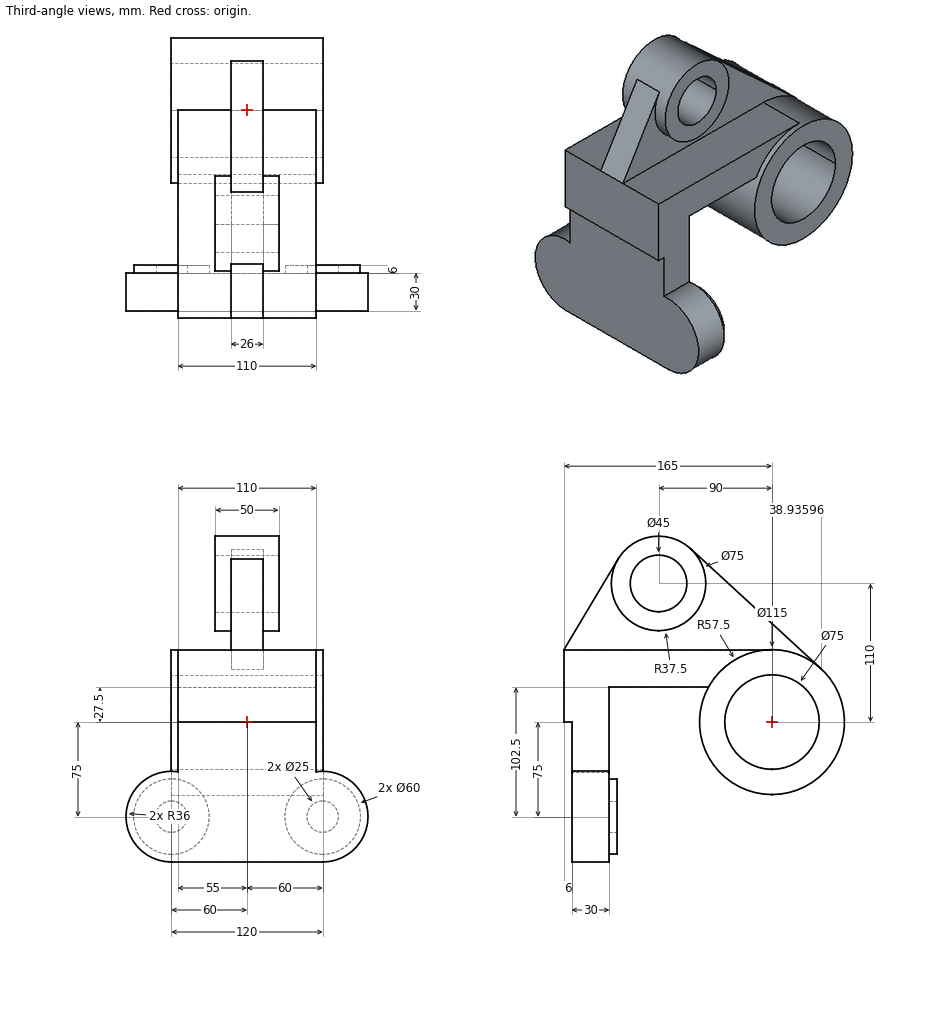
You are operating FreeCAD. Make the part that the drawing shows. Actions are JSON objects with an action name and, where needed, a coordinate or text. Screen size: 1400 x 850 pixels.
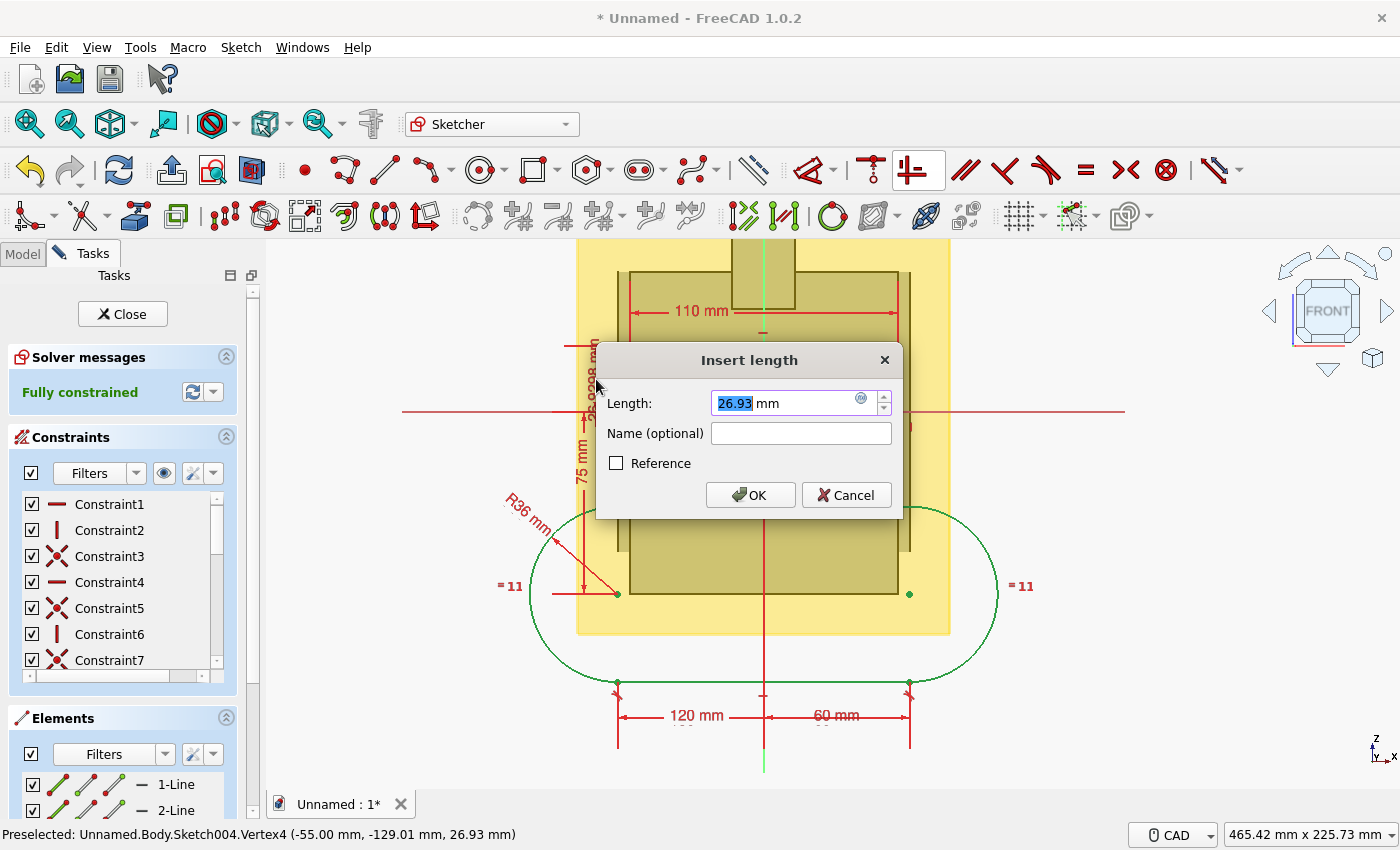
{"action": "type", "text": "27.5"}
{"action": "key", "text": "Return"}
{"action": "key", "text": "Escape"}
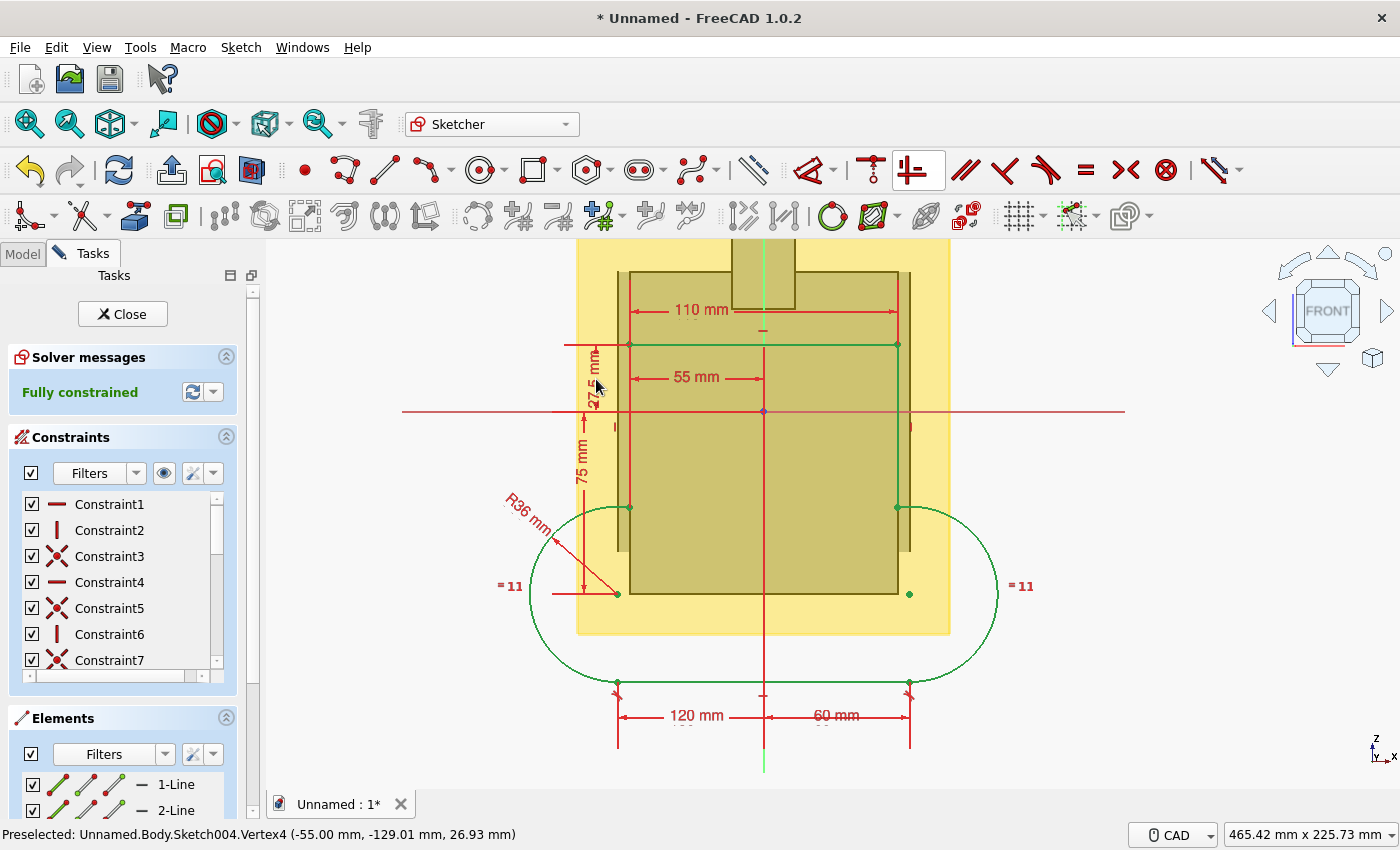
{"action": "left_click", "coordinate": [123, 314]}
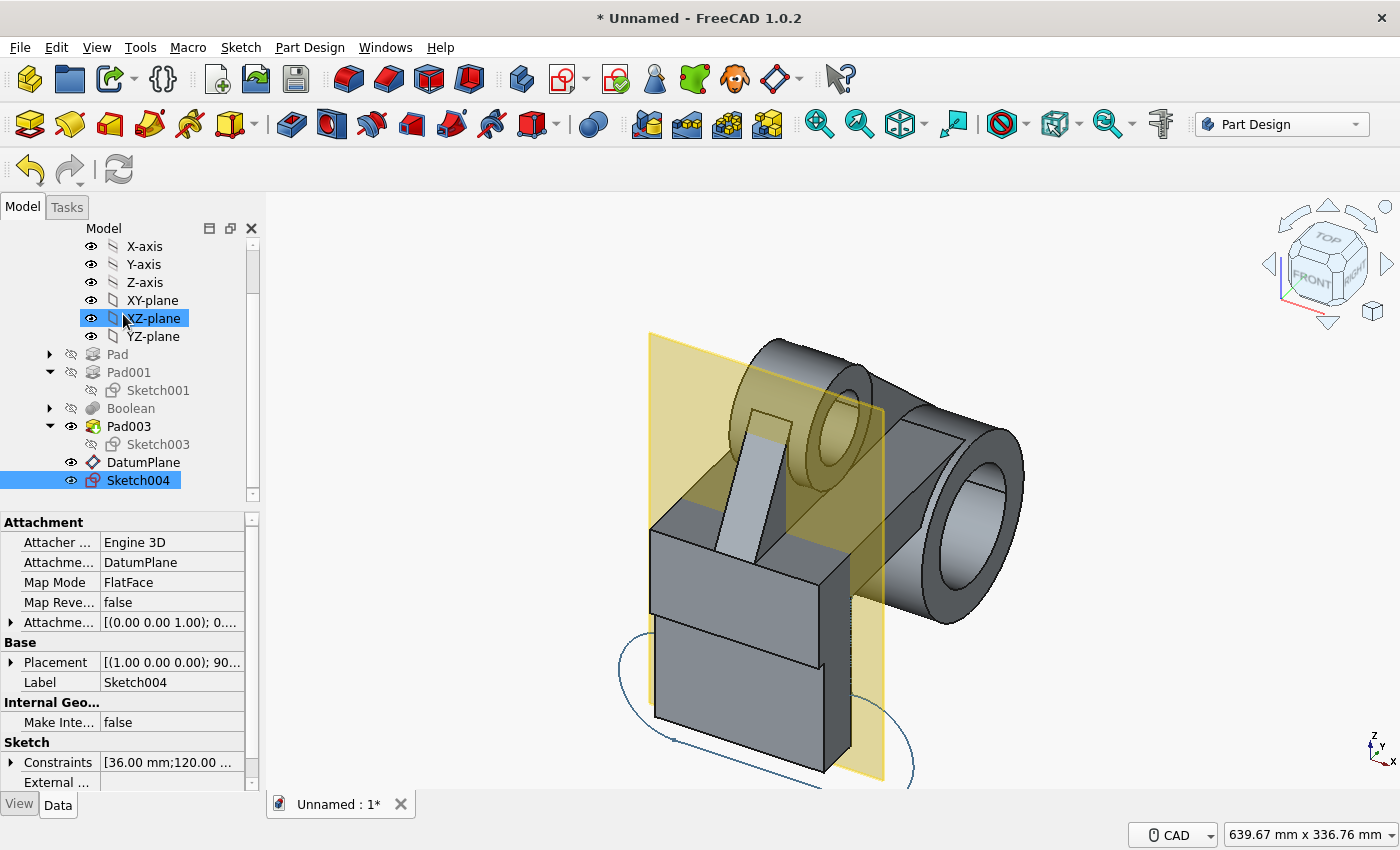
{"action": "left_click", "coordinate": [30, 124]}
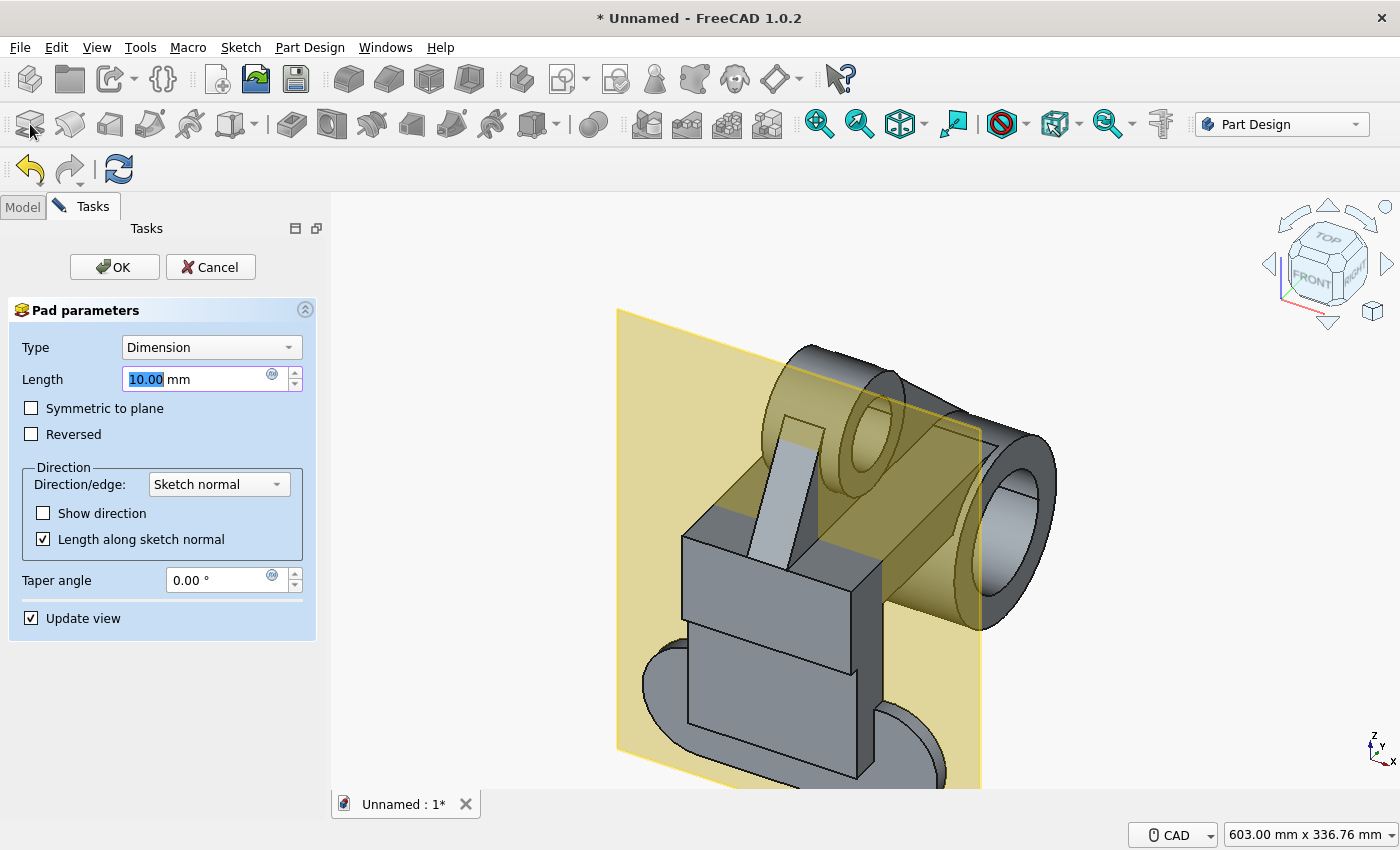
{"action": "type", "text": "30"}
{"action": "key", "text": "Tab"}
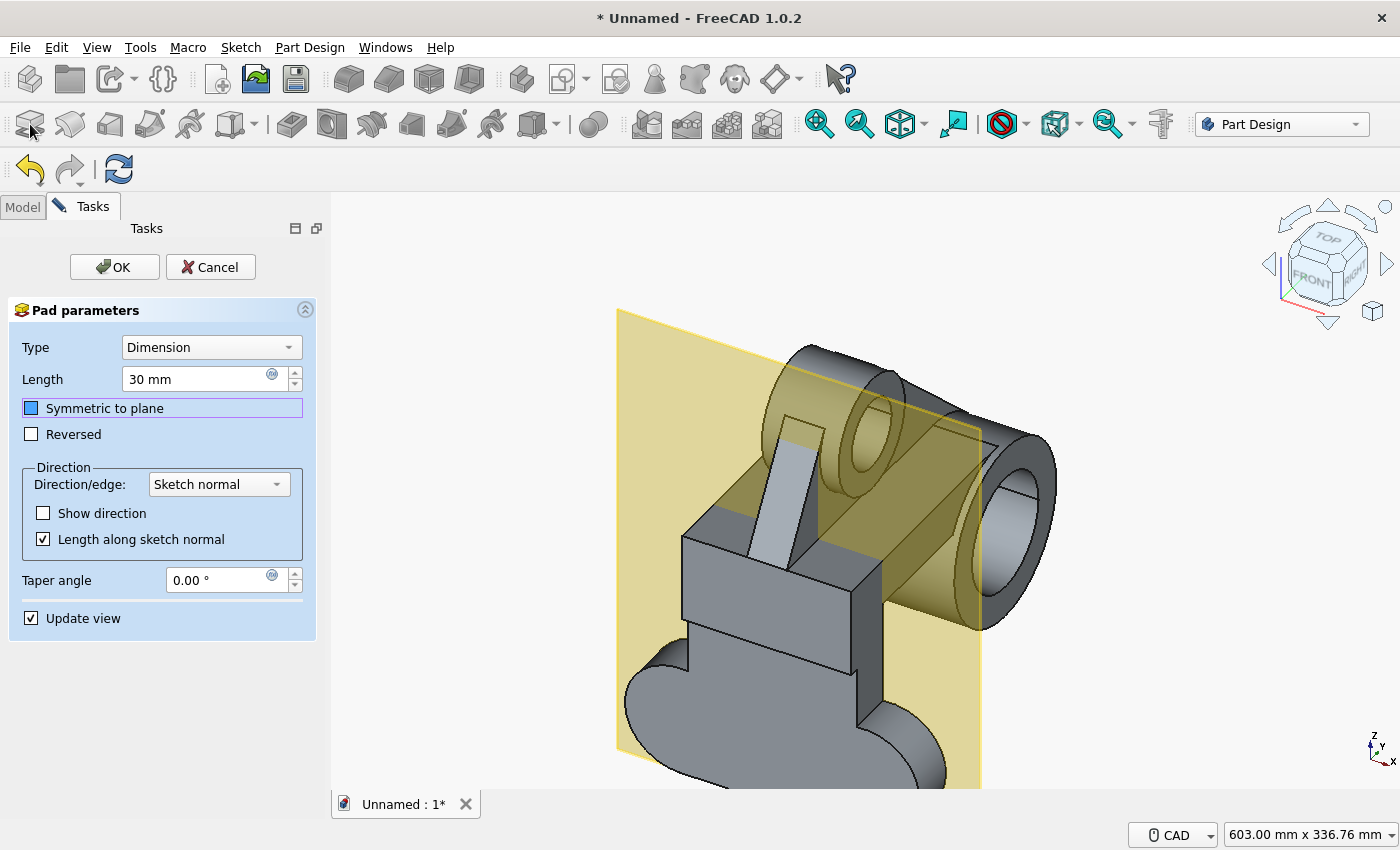
{"action": "left_click", "coordinate": [115, 267]}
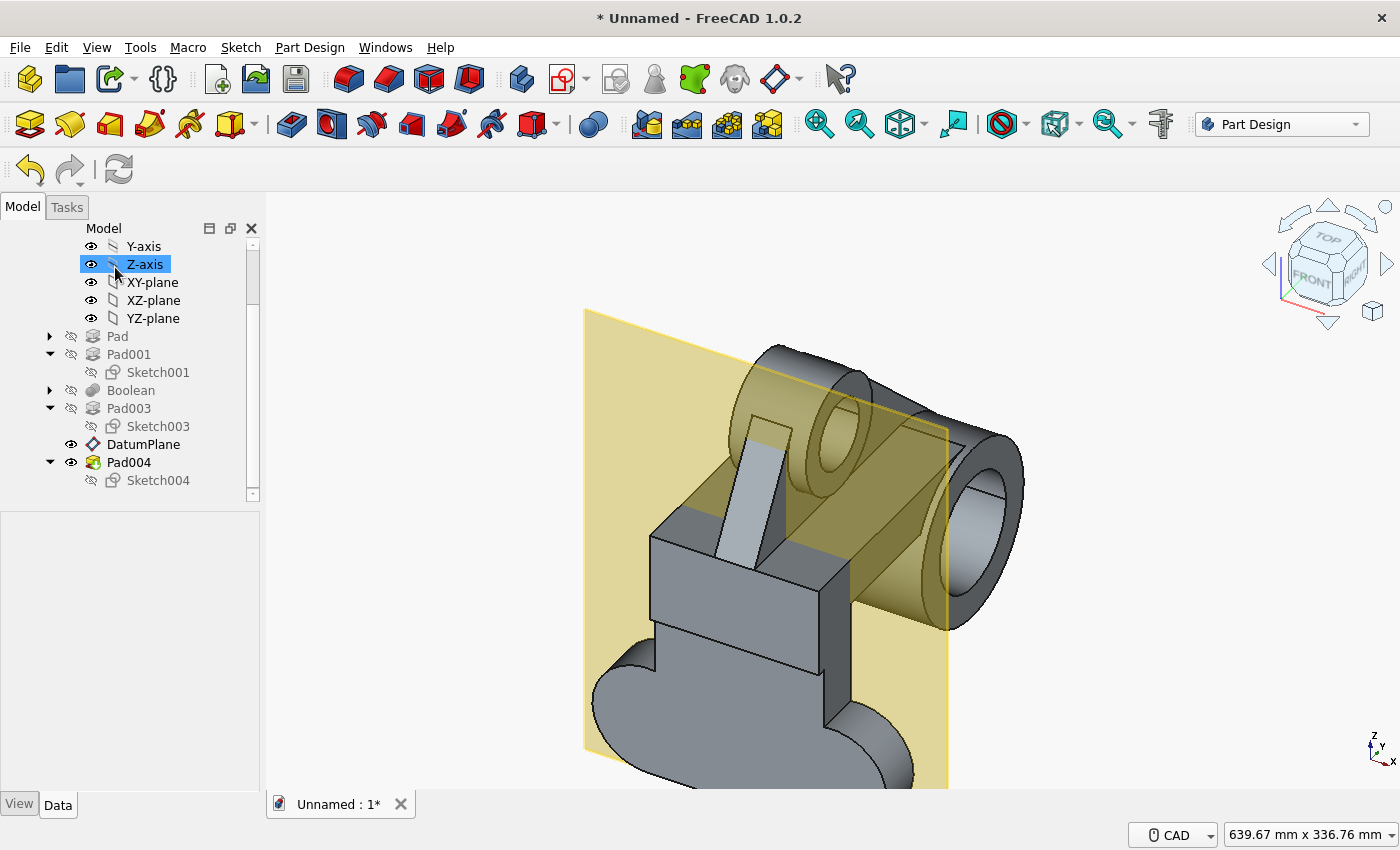
{"action": "left_click", "coordinate": [116, 444]}
{"action": "key", "text": "space"}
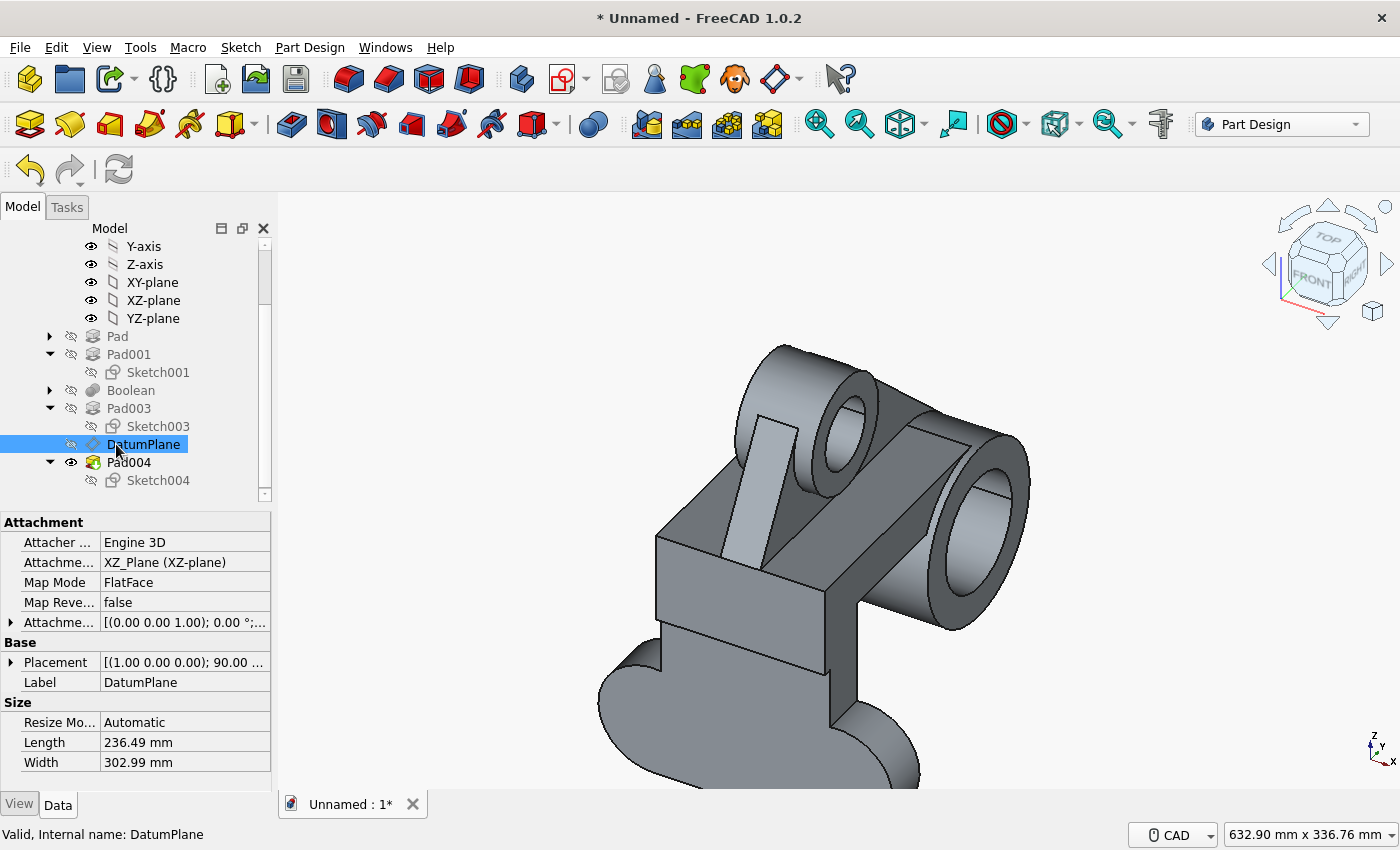
{"action": "key", "text": "v f"}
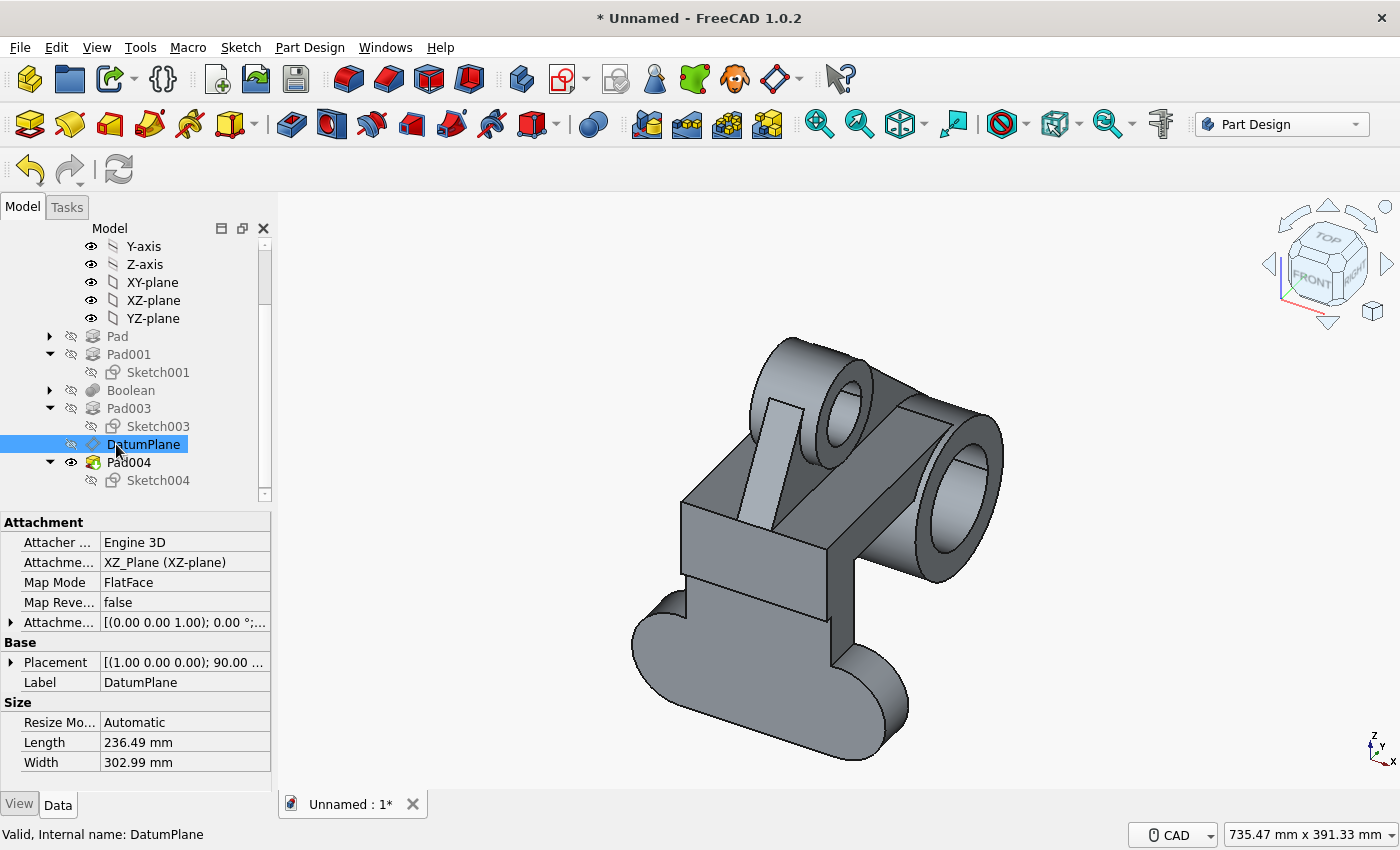
{"action": "key", "text": "4"}